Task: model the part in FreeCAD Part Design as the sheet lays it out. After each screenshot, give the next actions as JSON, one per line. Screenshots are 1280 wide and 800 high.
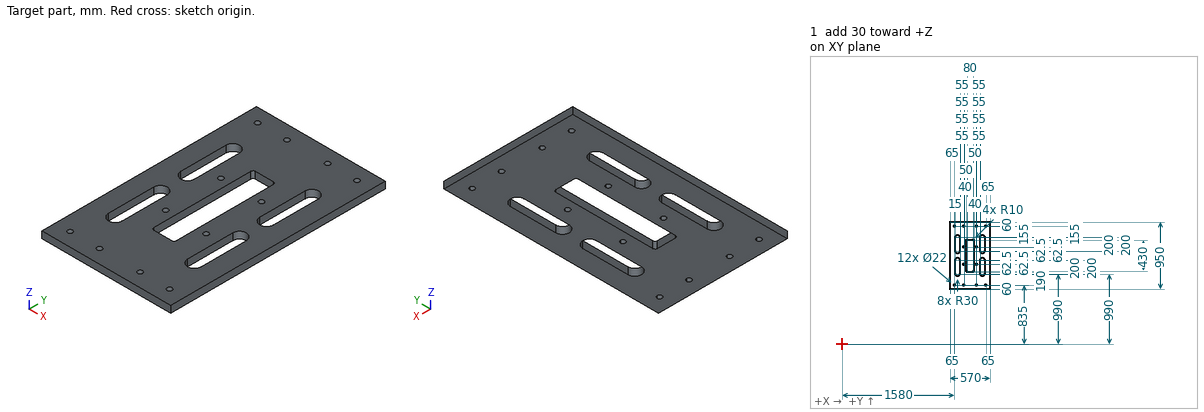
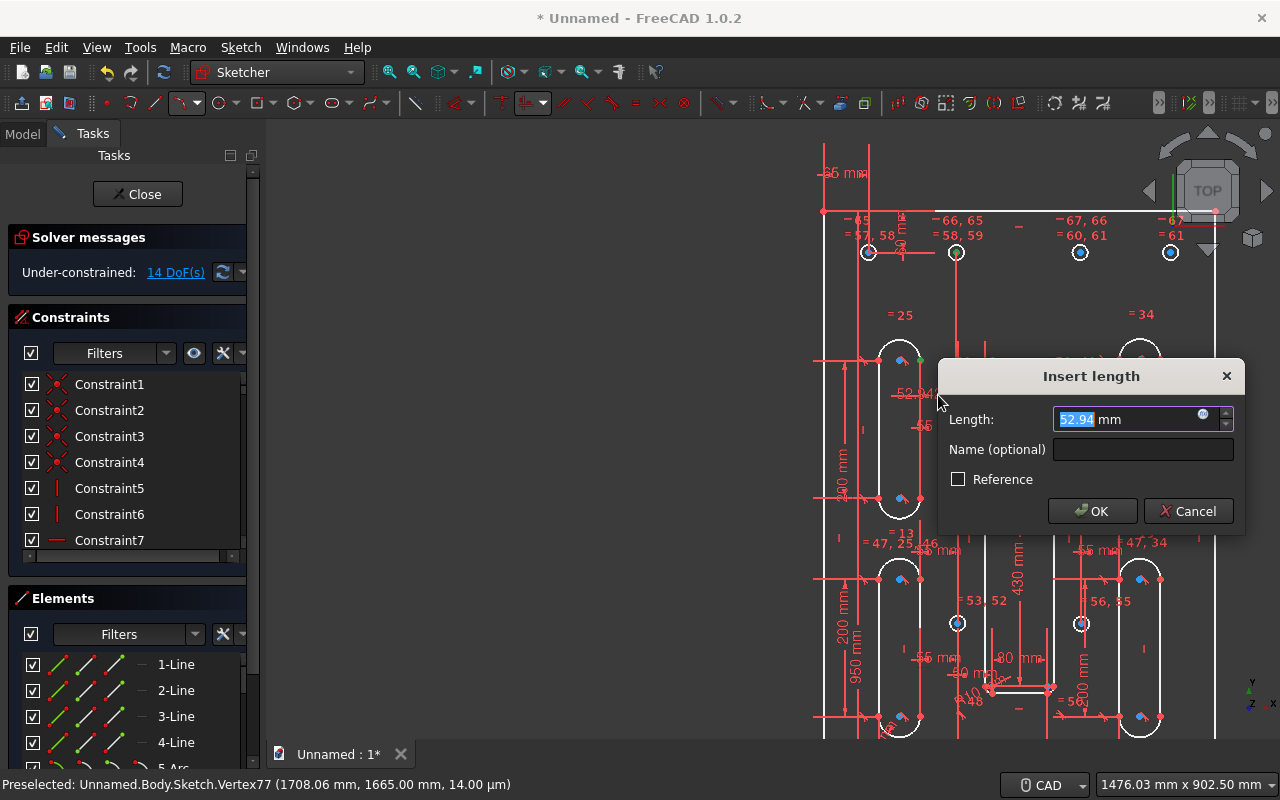
{"action": "type", "text": "55"}
{"action": "key", "text": "Return"}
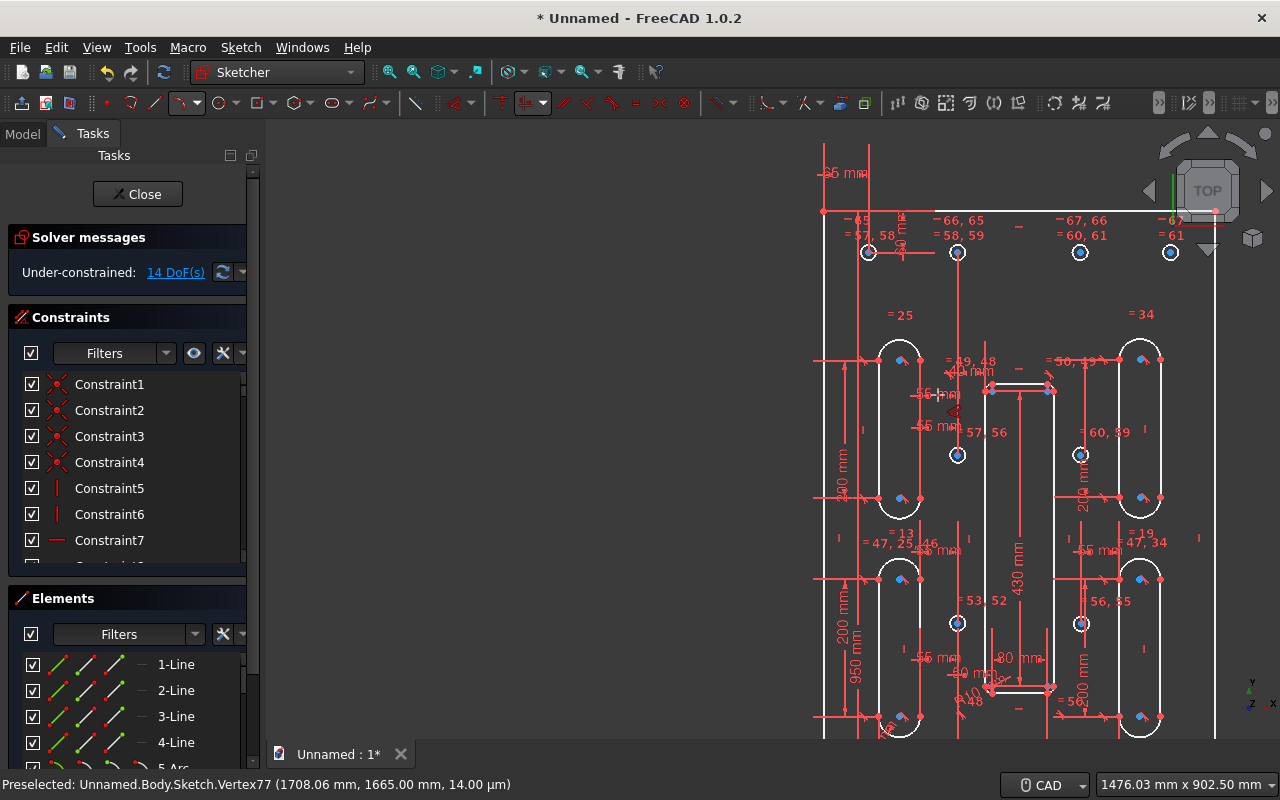
{"action": "scroll", "coordinate": [824, 211], "scroll_direction": "down", "scroll_amount": 5}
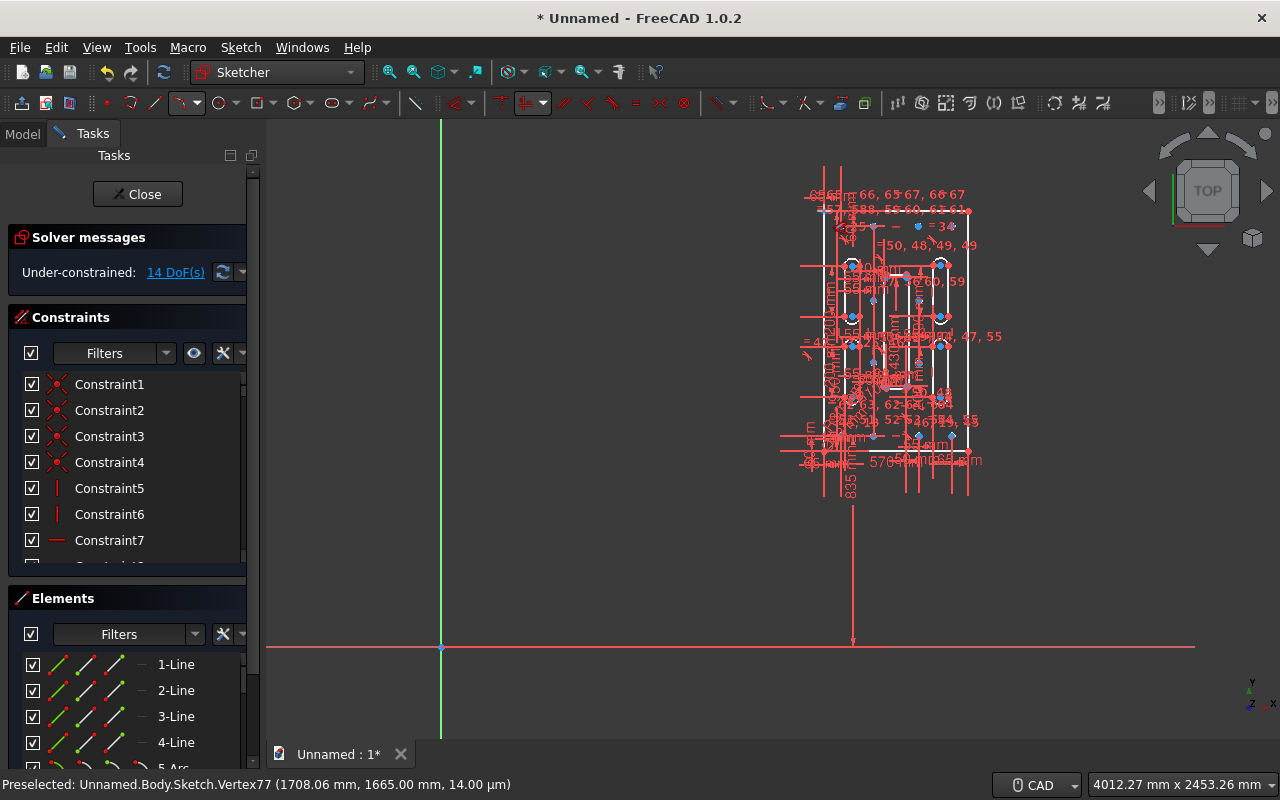
{"action": "scroll", "coordinate": [933, 316], "scroll_direction": "up", "scroll_amount": 6}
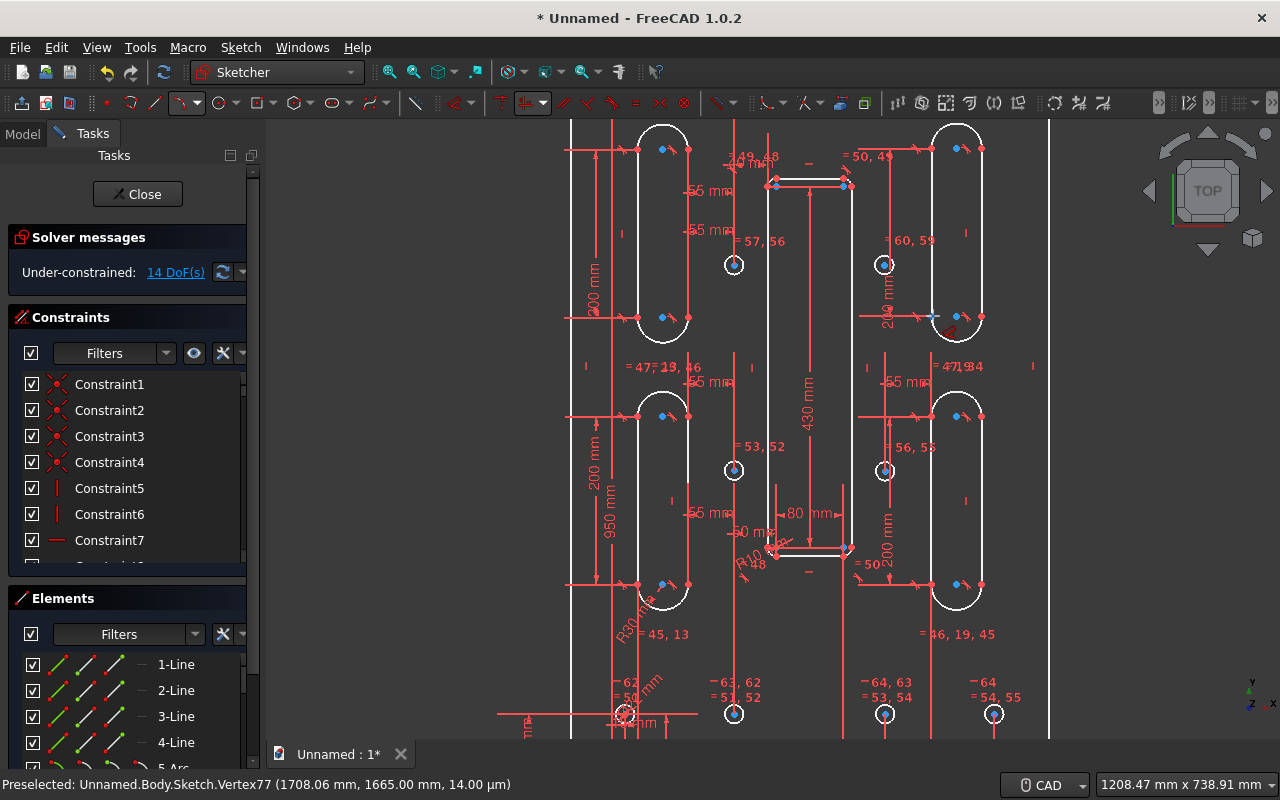
{"action": "left_click", "coordinate": [932, 316]}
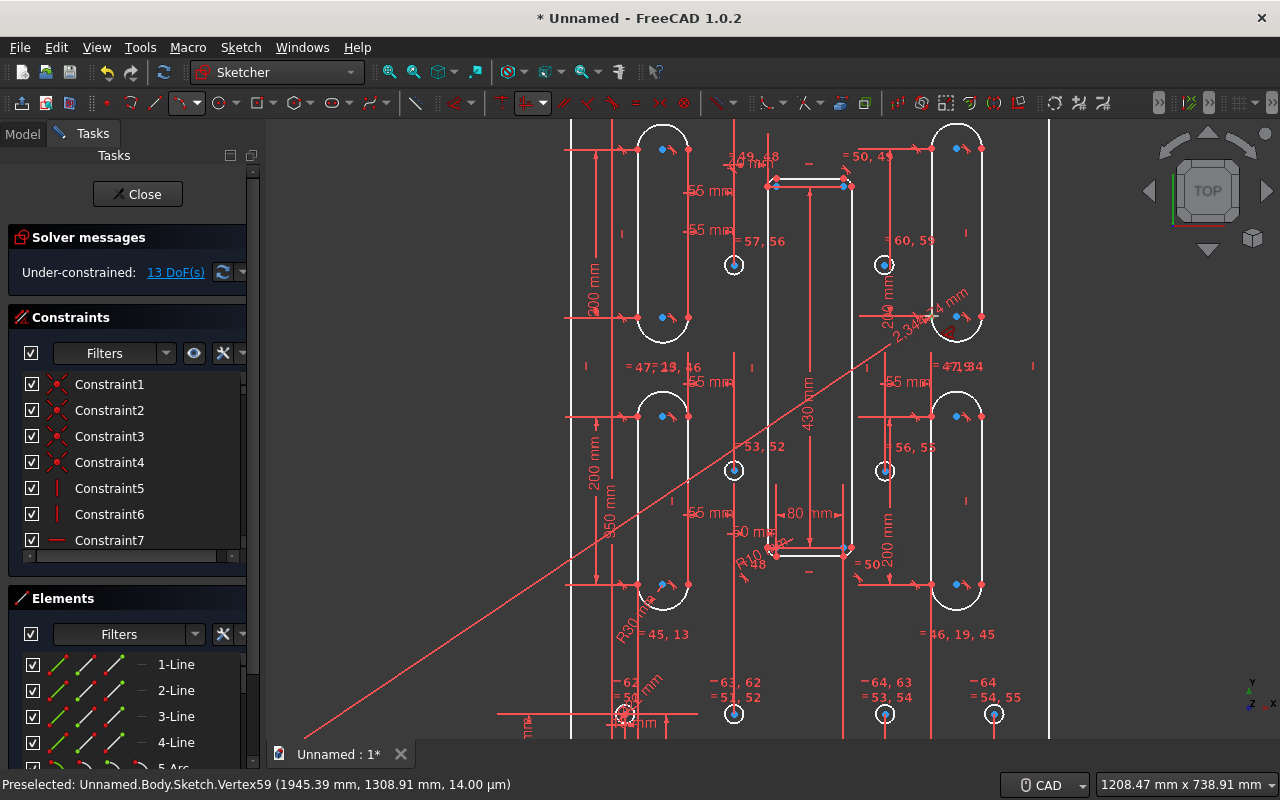
{"action": "left_click", "coordinate": [884, 265]}
{"action": "left_click", "coordinate": [908, 231]}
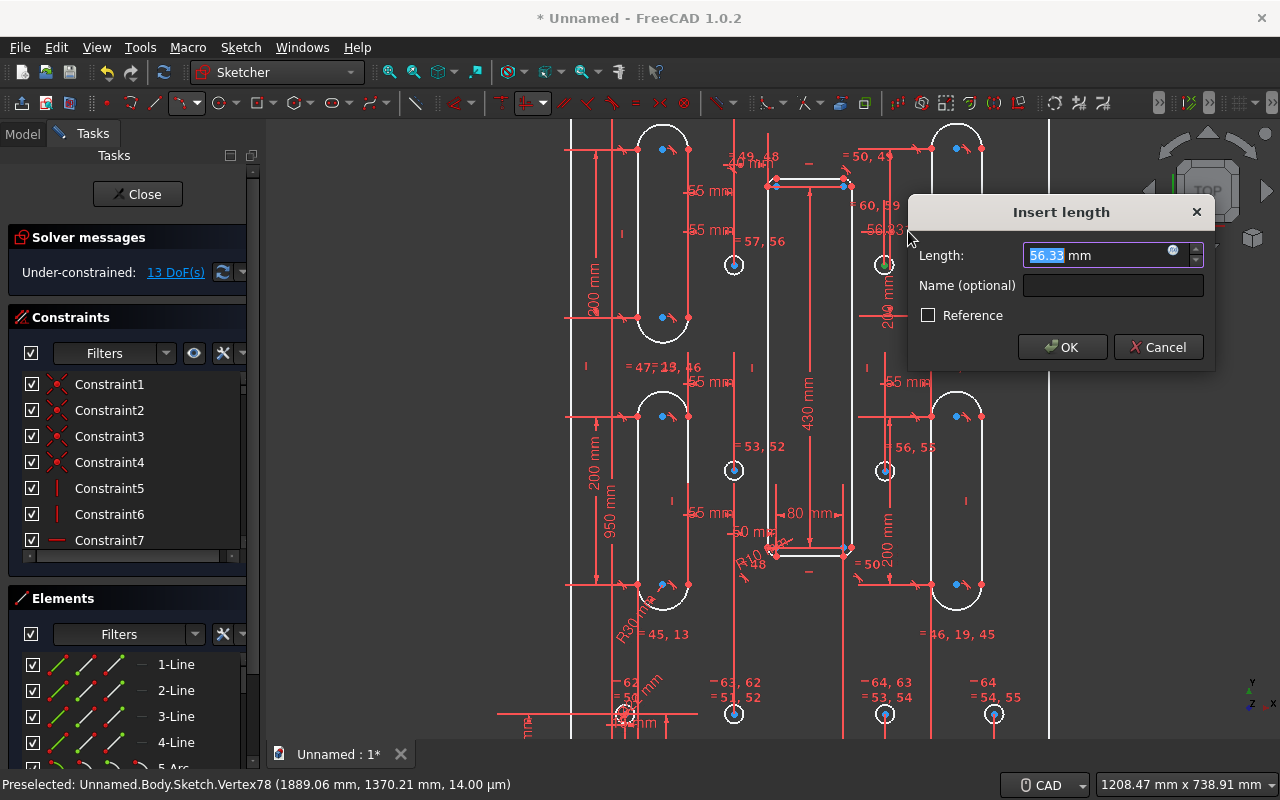
{"action": "type", "text": "55"}
{"action": "key", "text": "Return"}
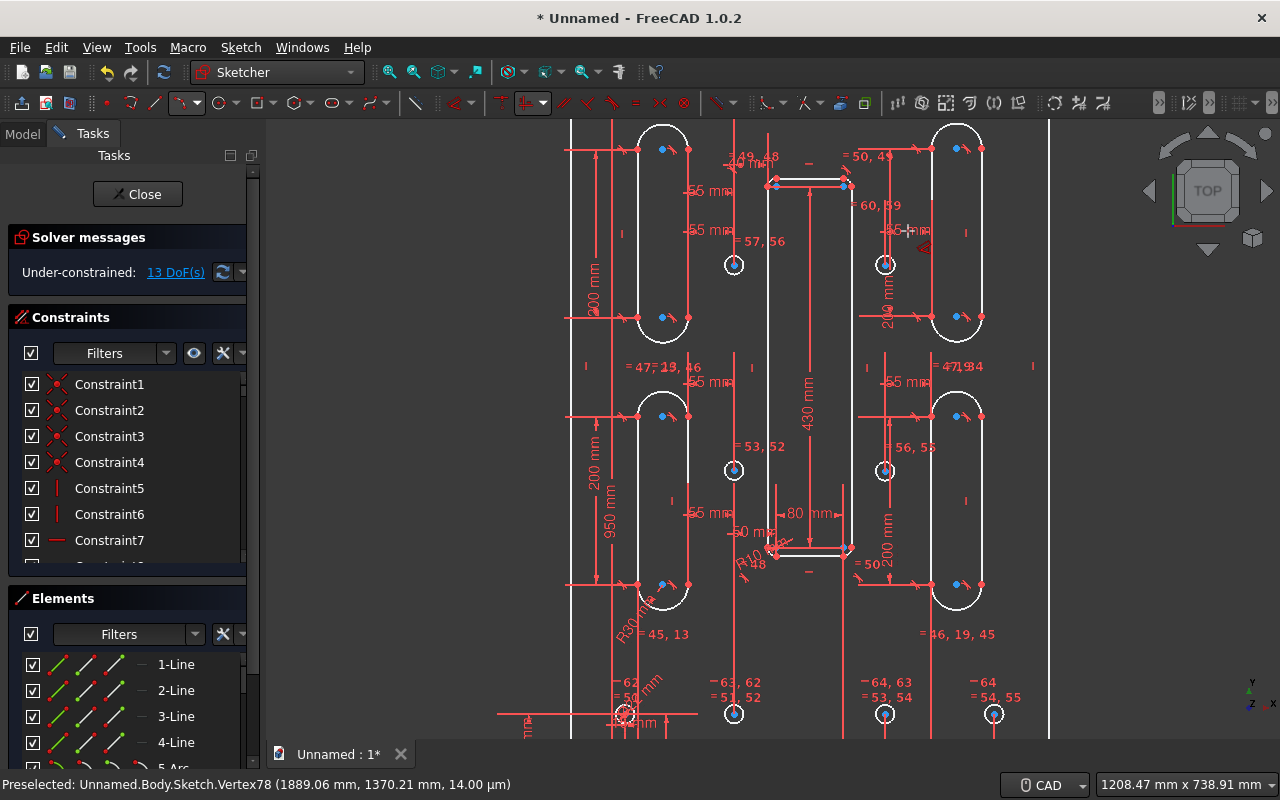
{"action": "scroll", "coordinate": [852, 187], "scroll_direction": "up", "scroll_amount": 2}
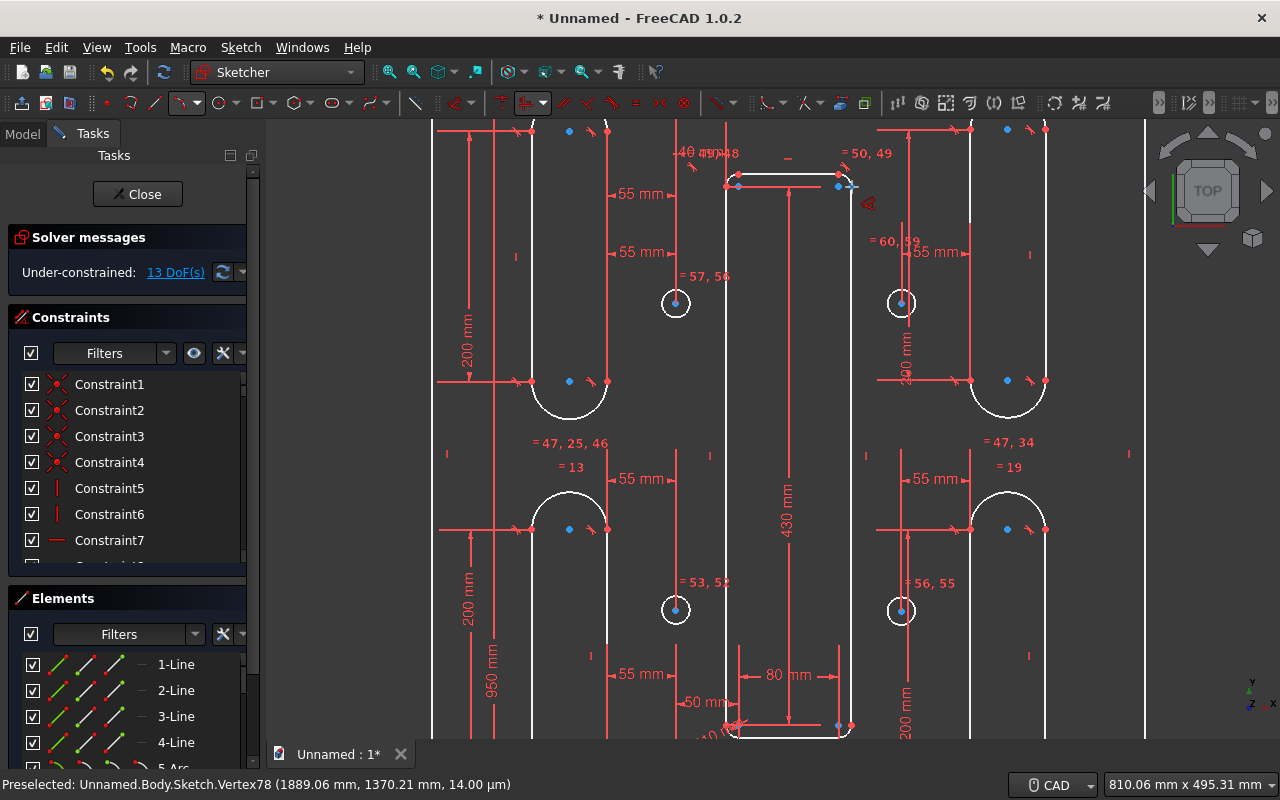
{"action": "left_click", "coordinate": [851, 187]}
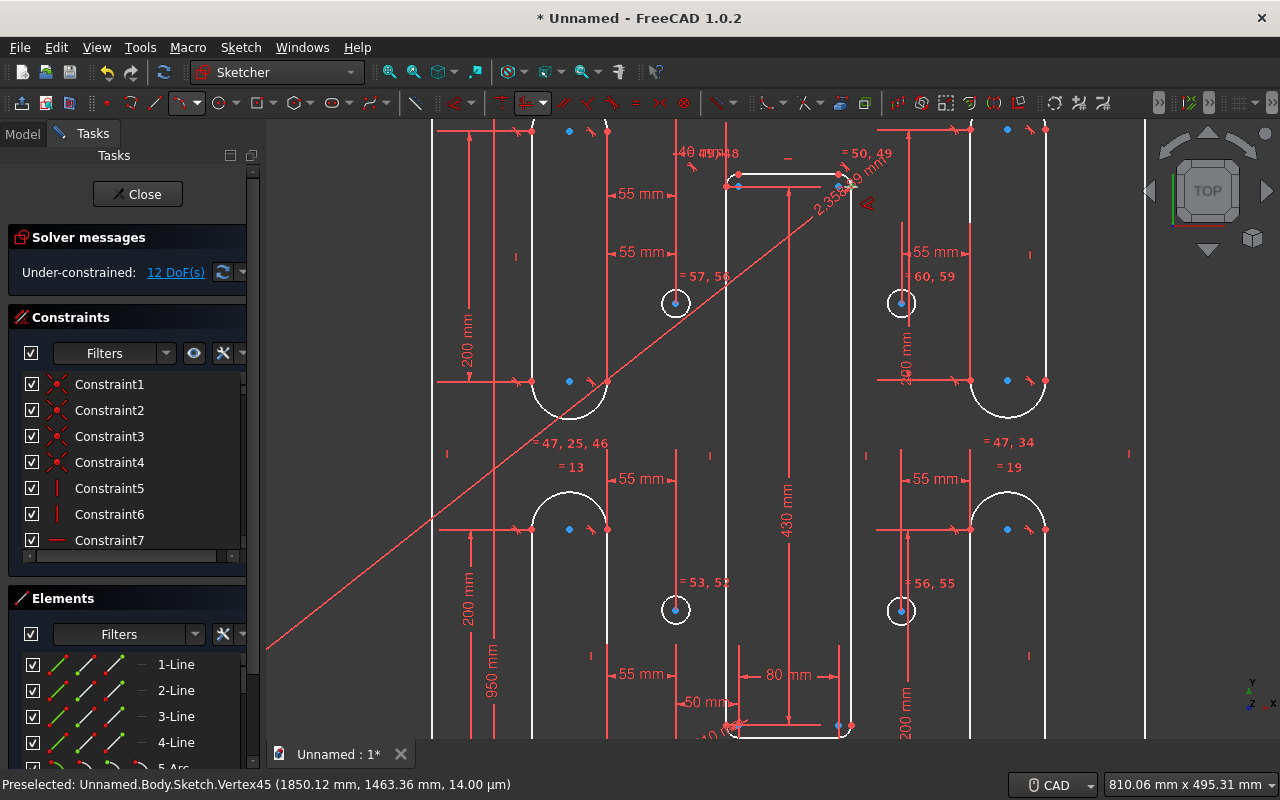
{"action": "left_click", "coordinate": [902, 303]}
{"action": "left_click", "coordinate": [876, 153]}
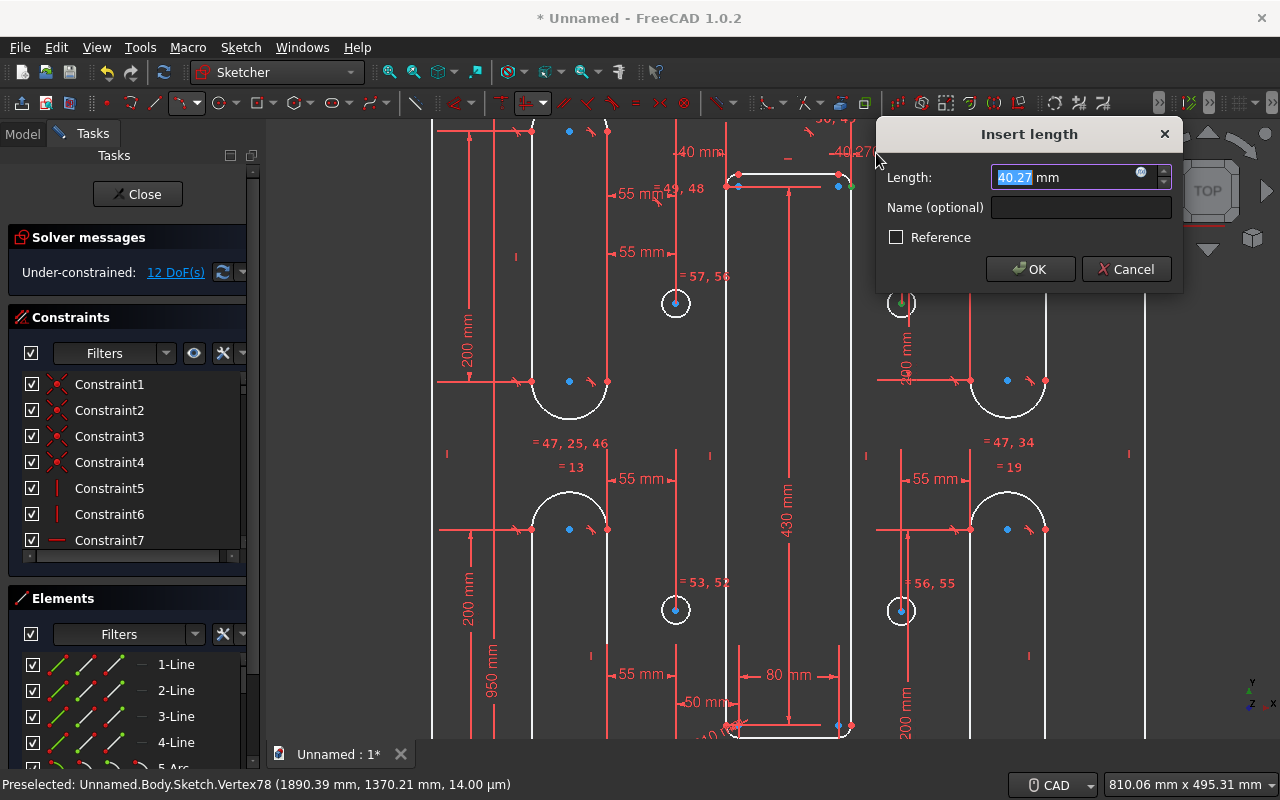
{"action": "type", "text": "40"}
{"action": "key", "text": "Return"}